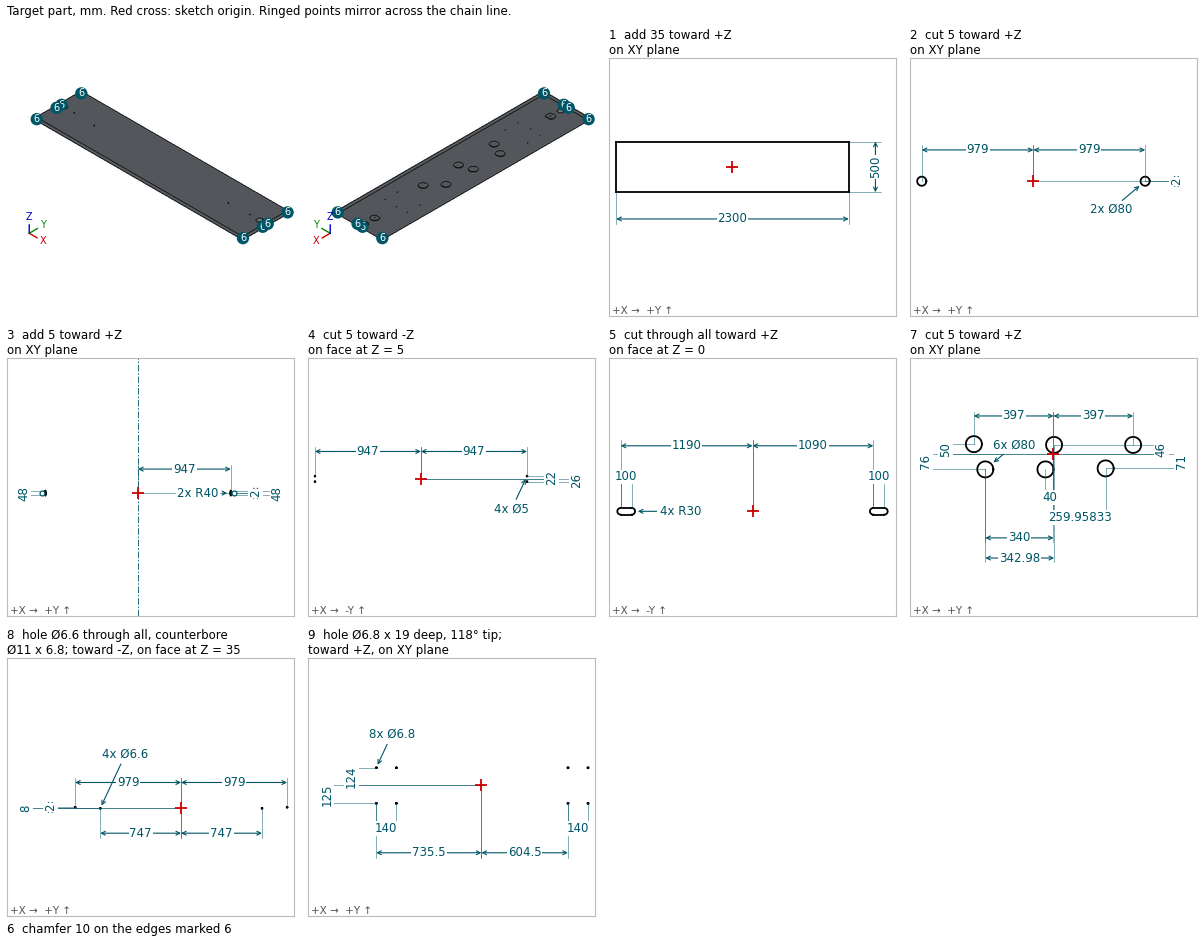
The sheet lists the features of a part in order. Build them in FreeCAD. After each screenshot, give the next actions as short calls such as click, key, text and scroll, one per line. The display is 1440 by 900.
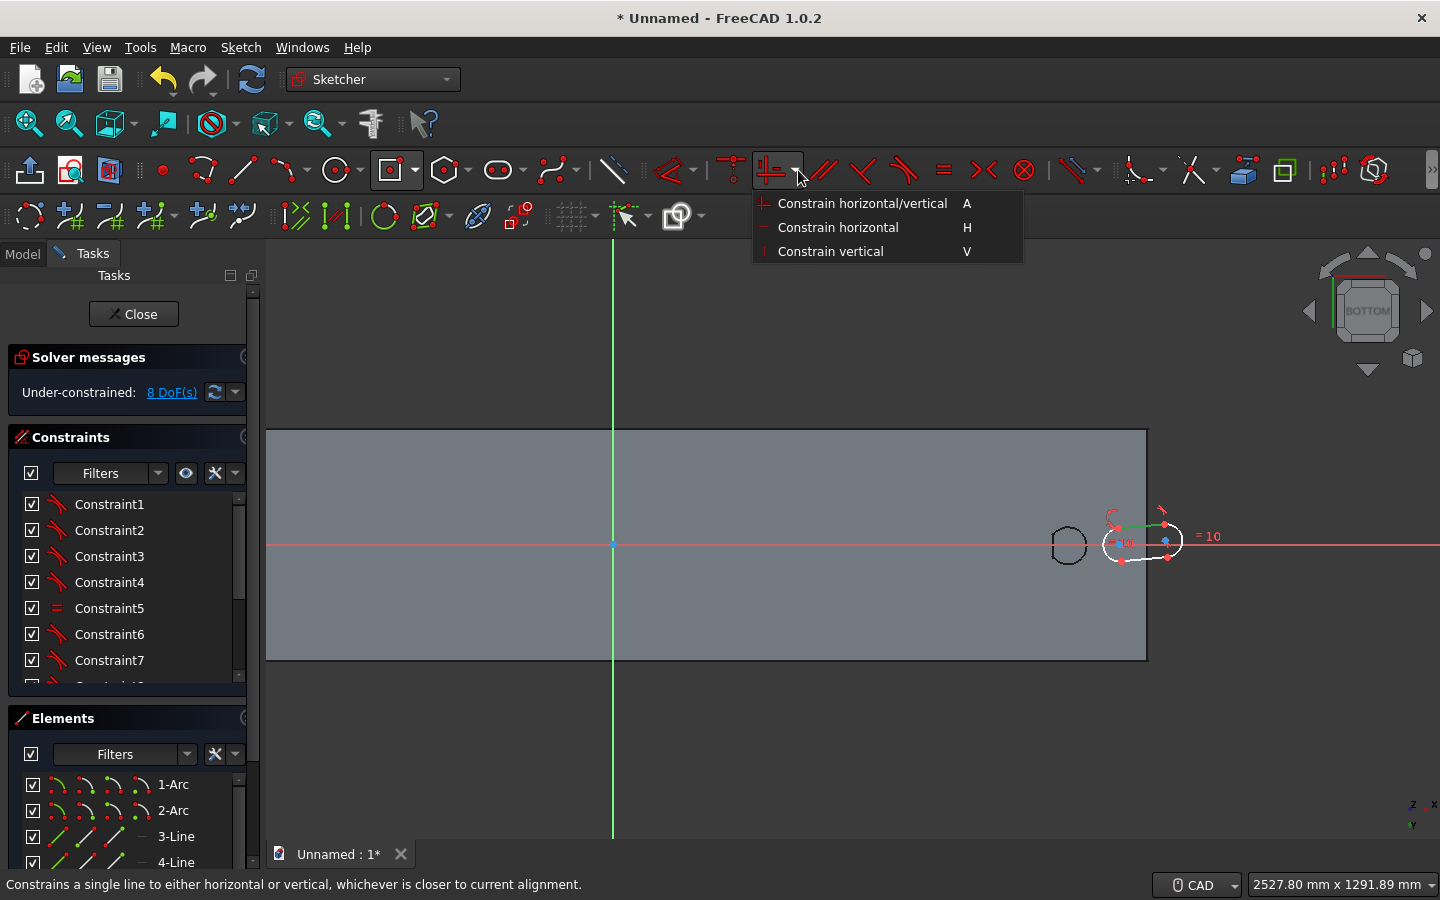
click(888, 227)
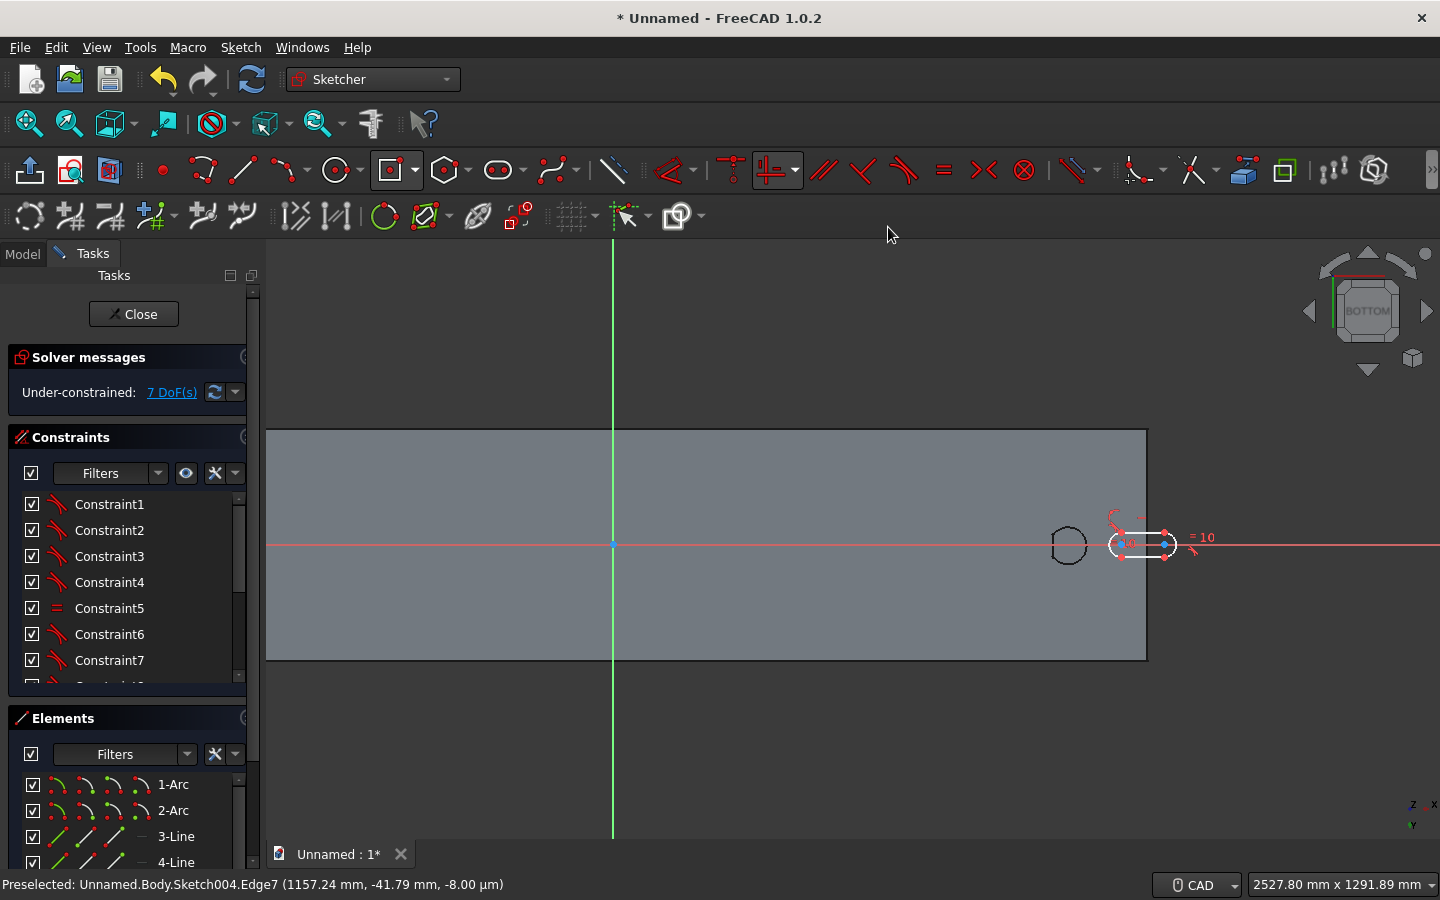
scroll(1132, 527, down, 2)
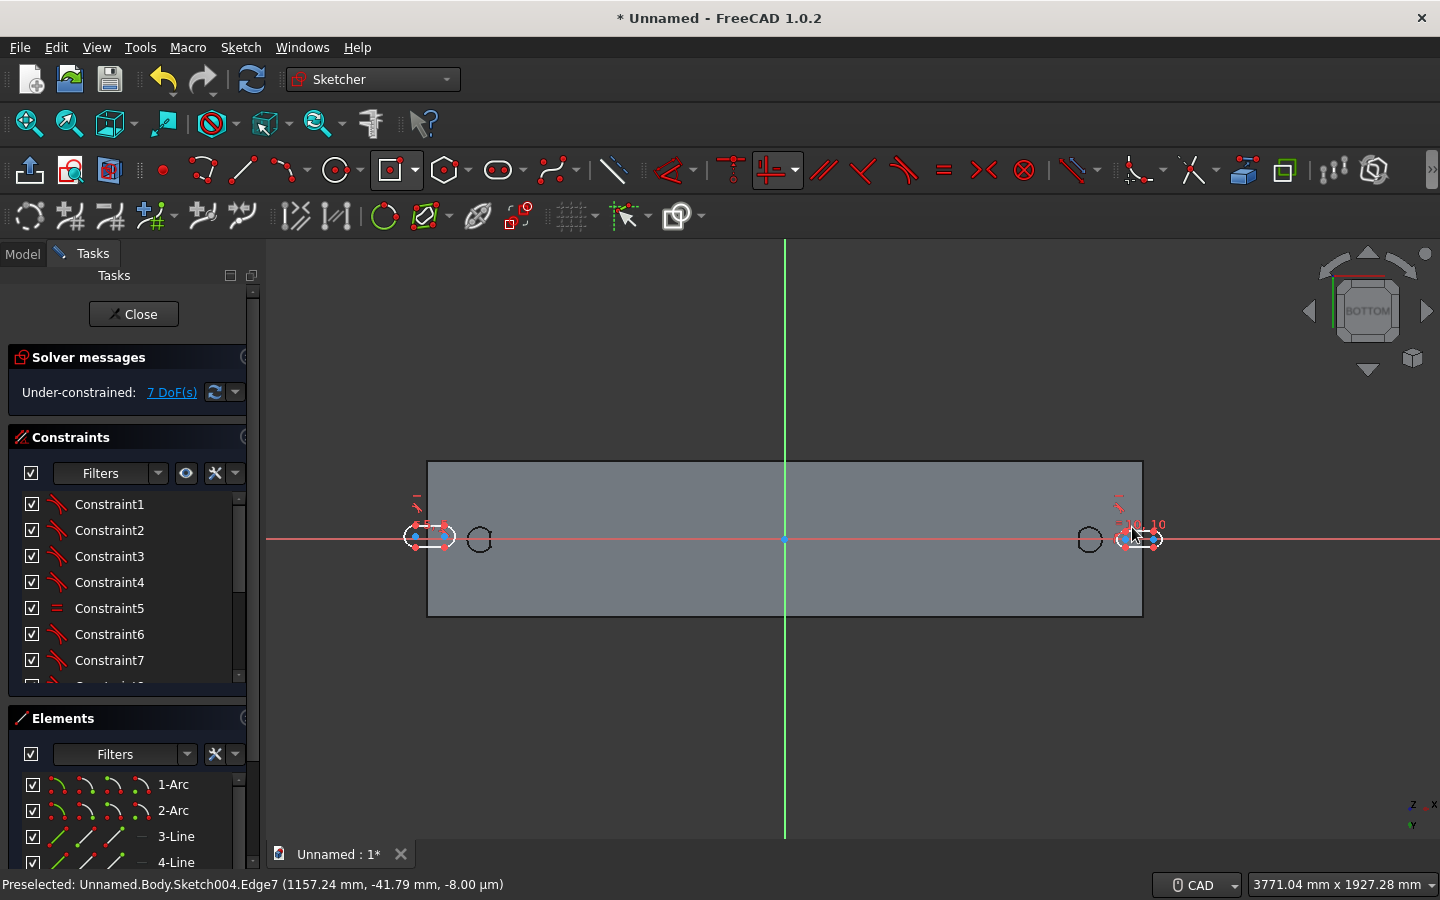
scroll(406, 530, up, 3)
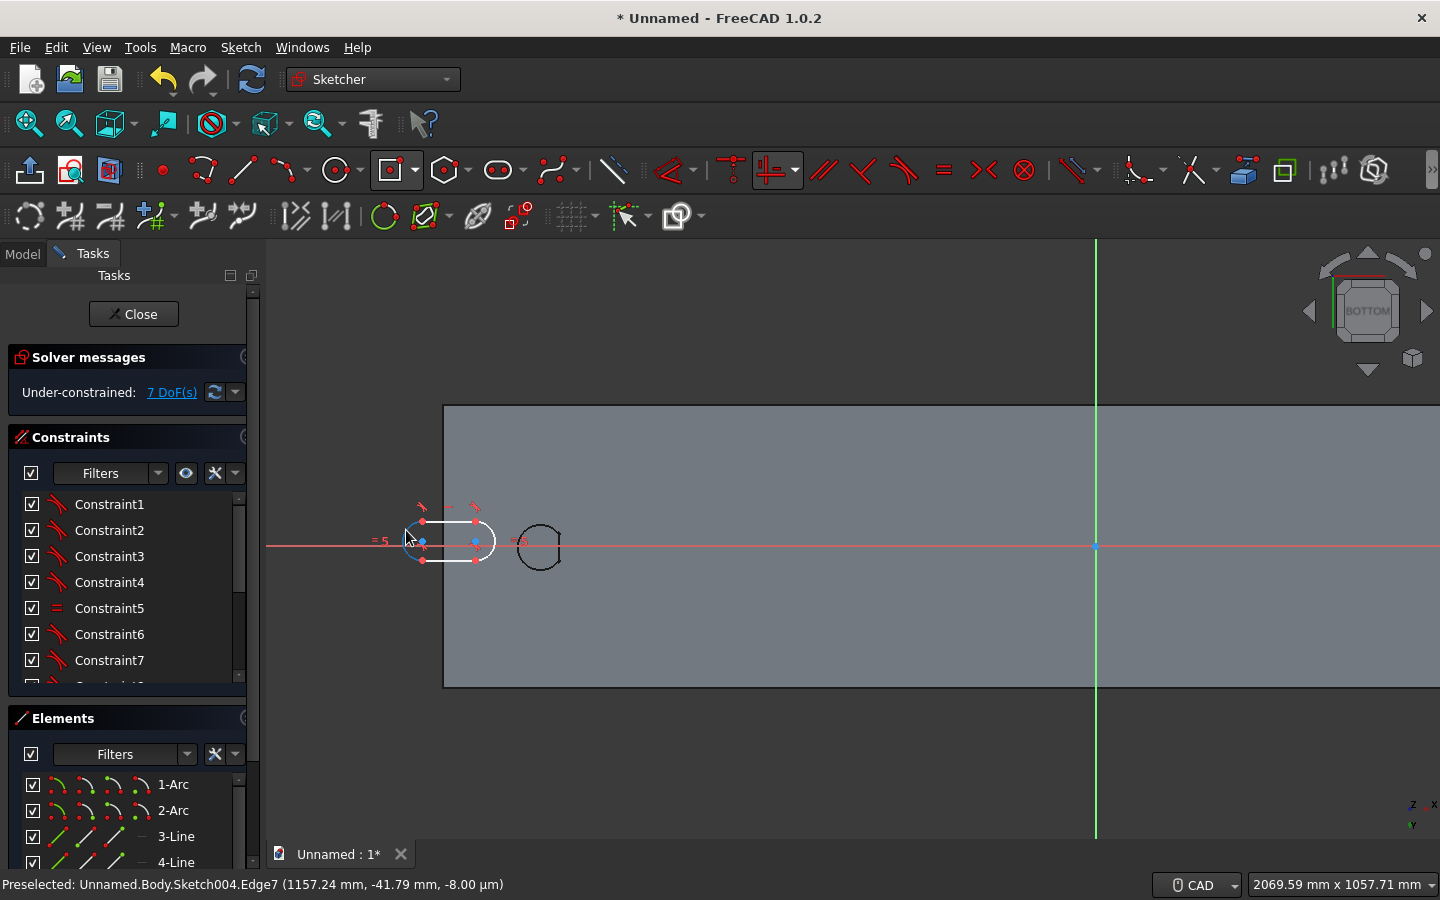
click(407, 530)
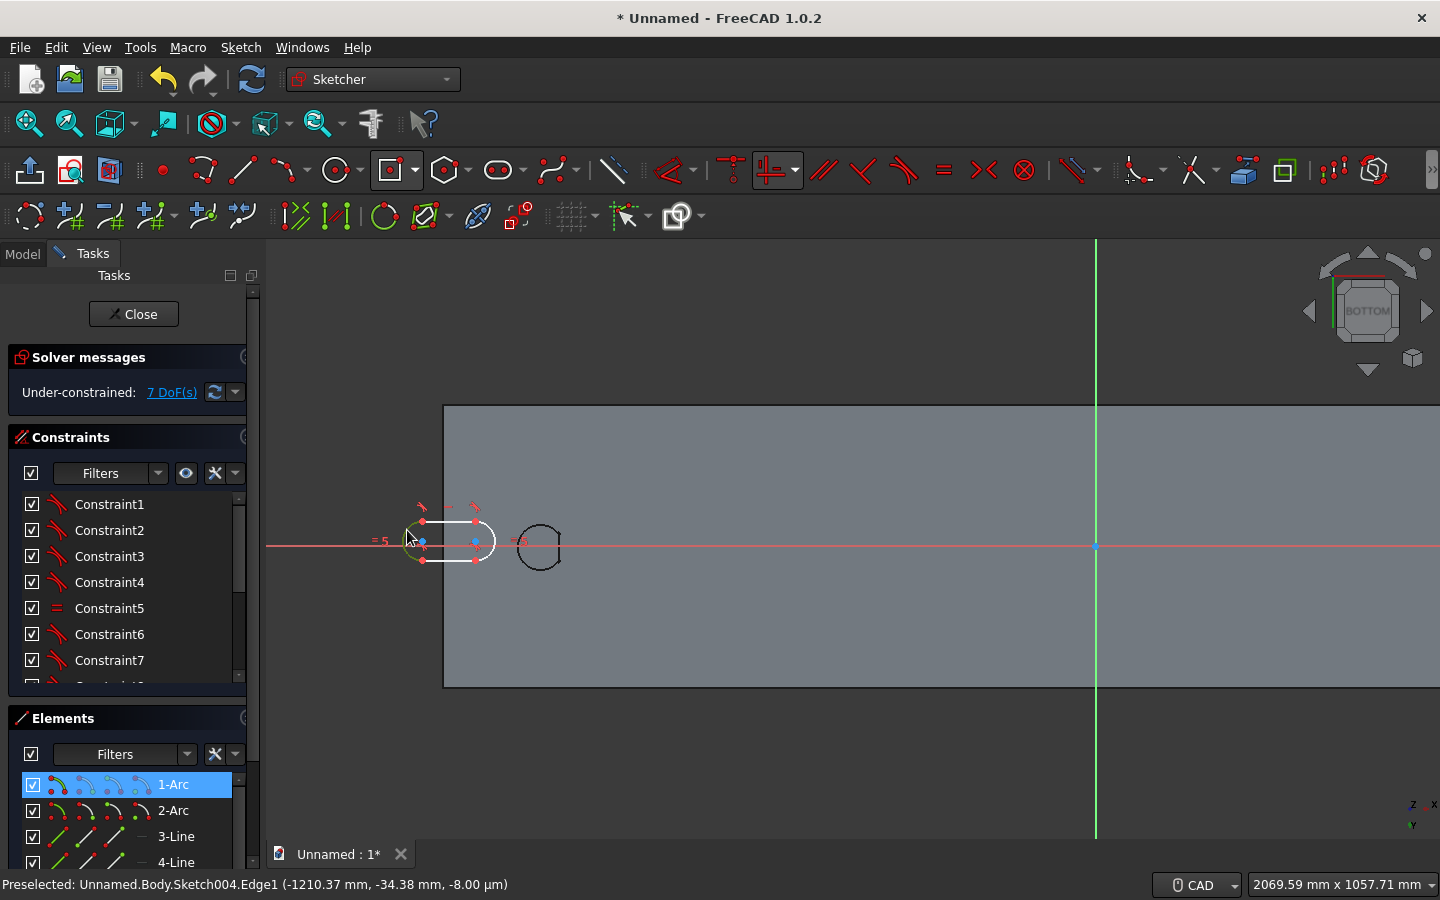
scroll(406, 530, down, 3)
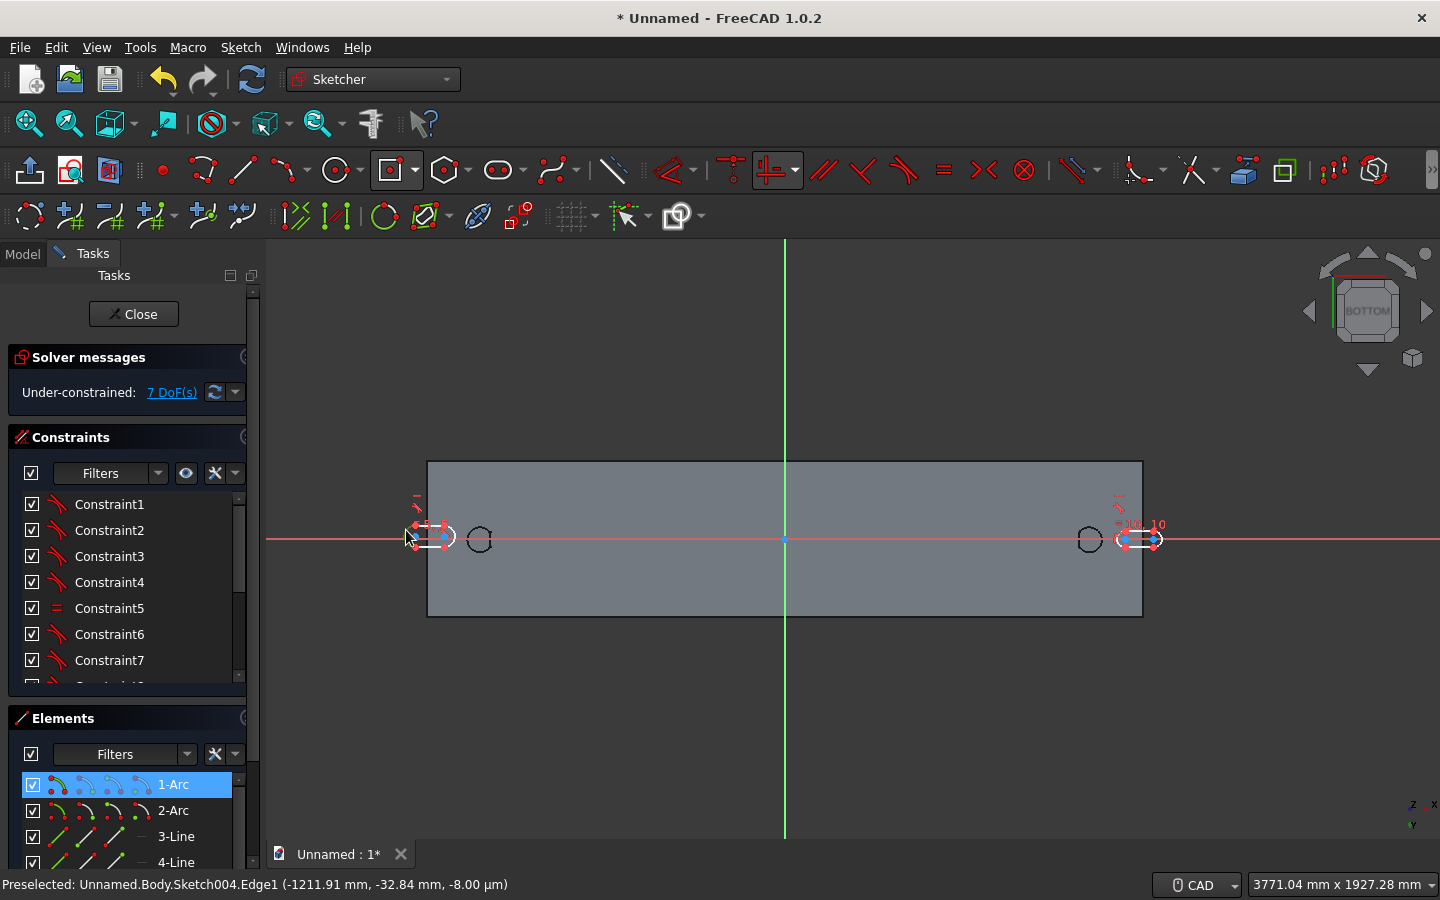
scroll(1117, 539, up, 3)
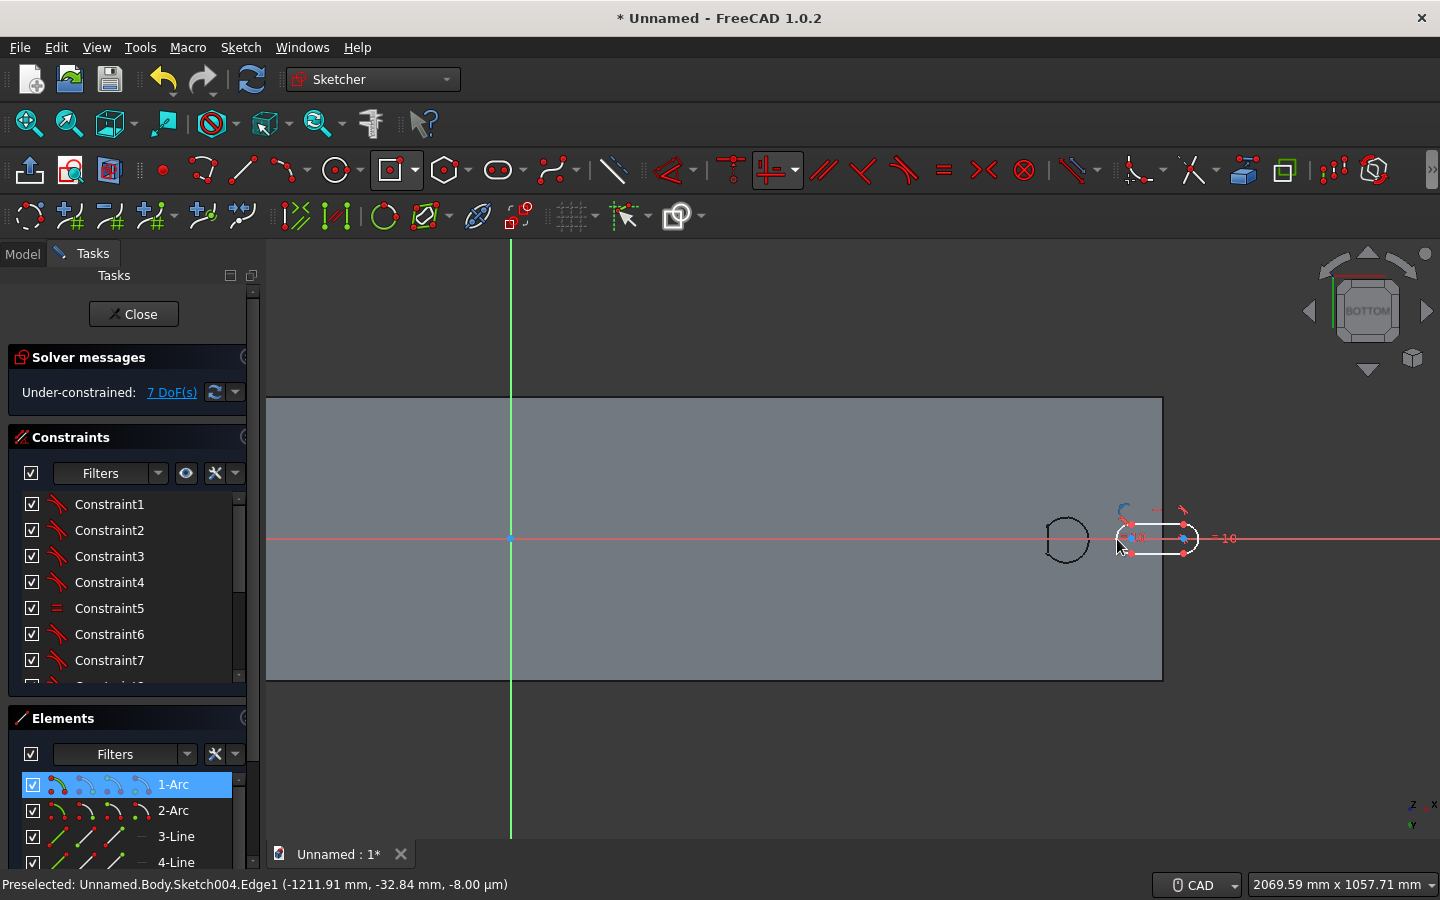
click(1116, 539)